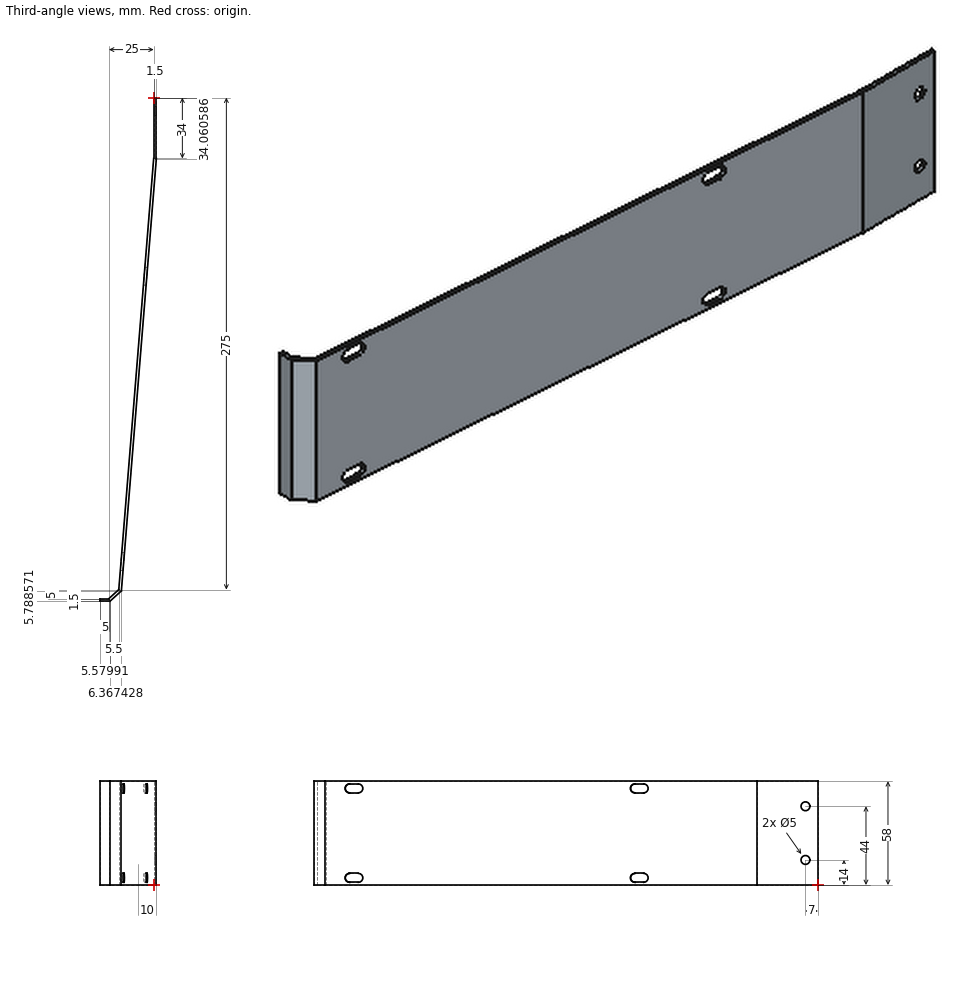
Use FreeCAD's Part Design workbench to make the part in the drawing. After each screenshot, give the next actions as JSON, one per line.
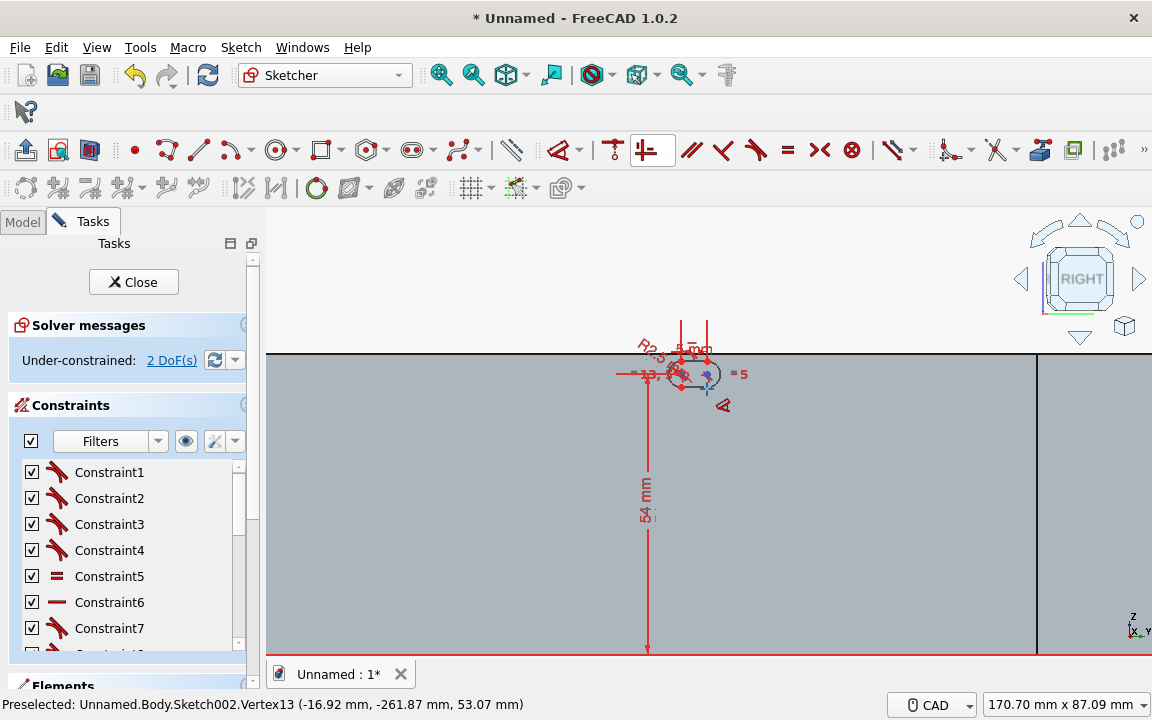
{"action": "left_click", "coordinate": [707, 387]}
{"action": "left_click", "coordinate": [847, 353]}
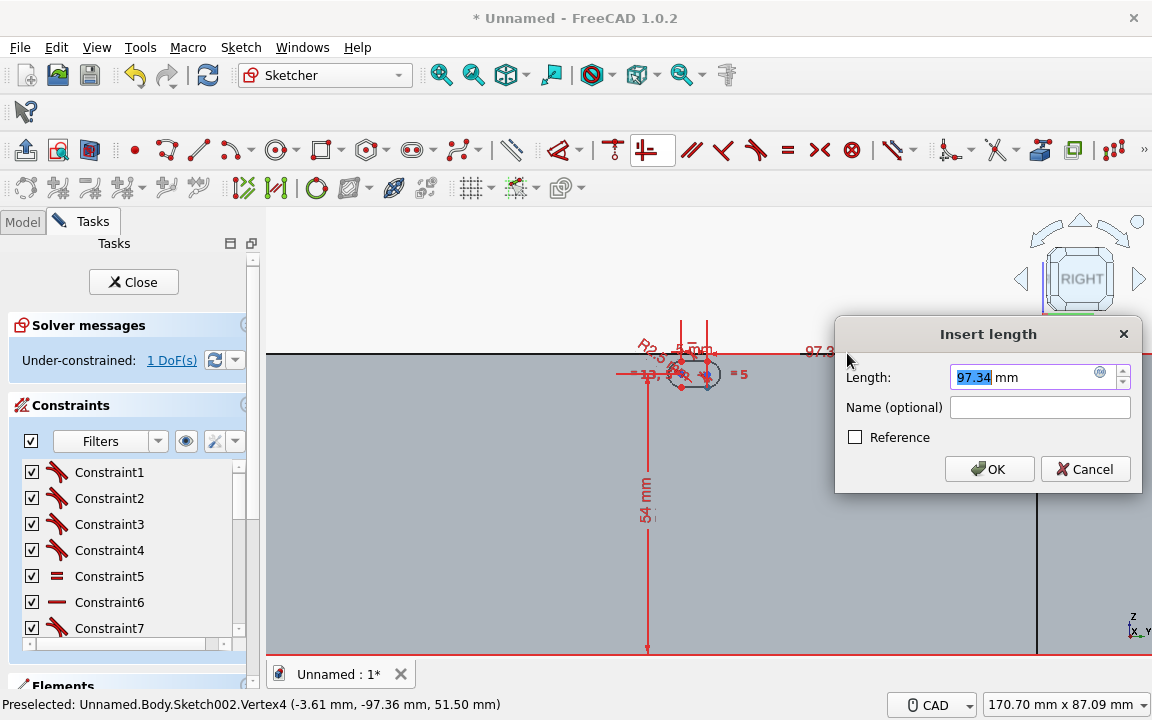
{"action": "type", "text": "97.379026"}
{"action": "key", "text": "Return"}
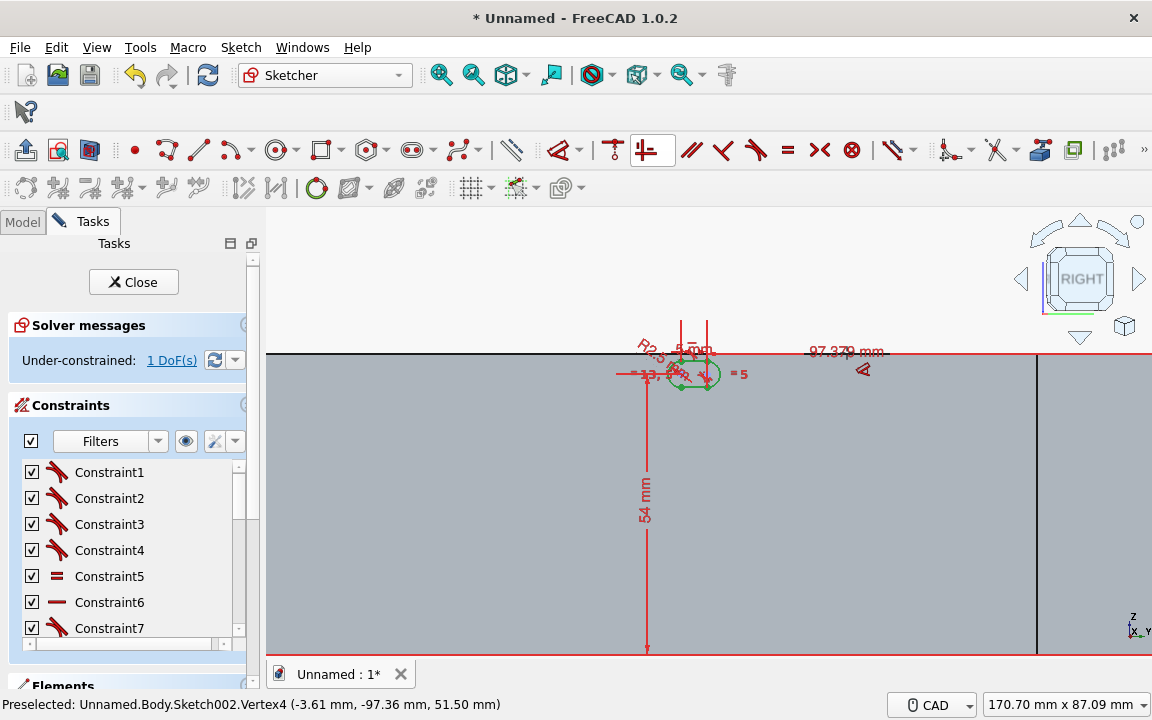
{"action": "scroll", "coordinate": [708, 389], "scroll_direction": "down", "scroll_amount": 5}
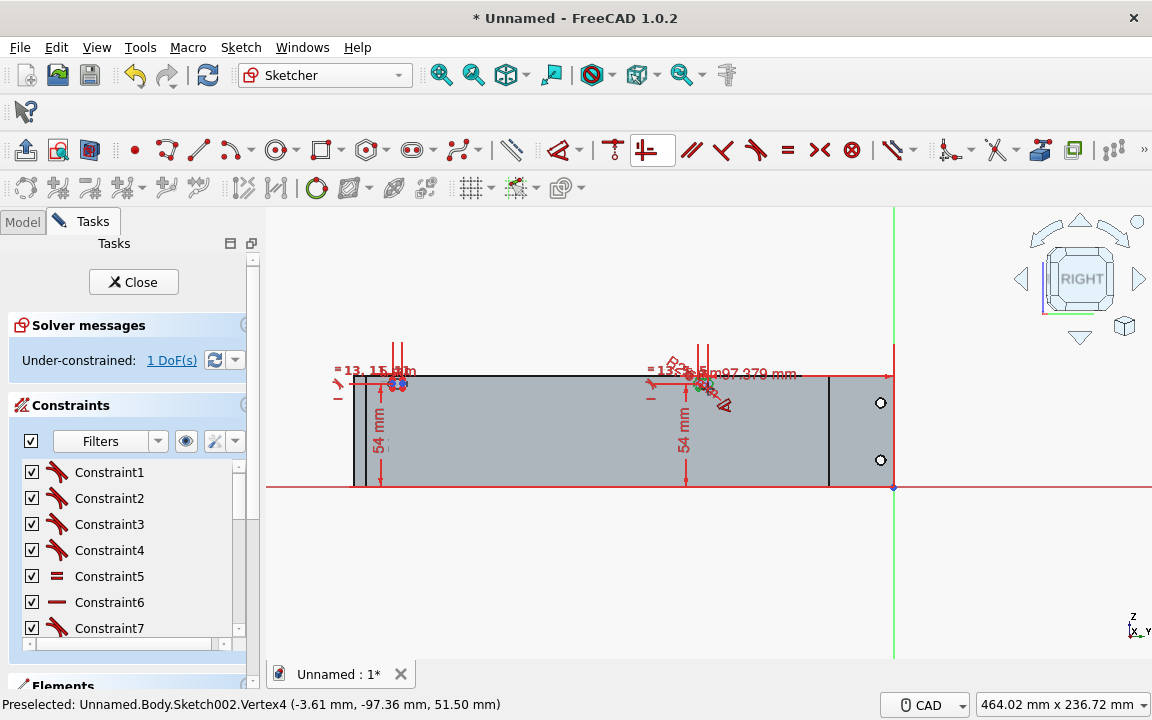
{"action": "scroll", "coordinate": [393, 379], "scroll_direction": "up", "scroll_amount": 5}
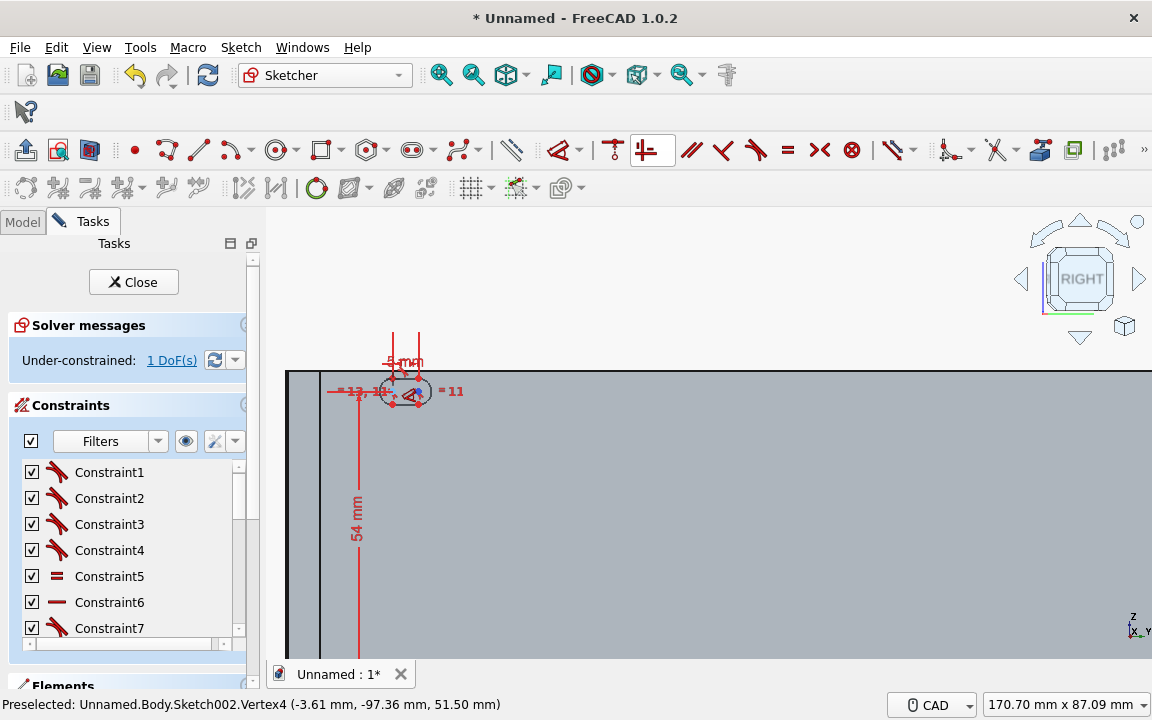
{"action": "left_click", "coordinate": [393, 379]}
{"action": "left_click", "coordinate": [690, 345]}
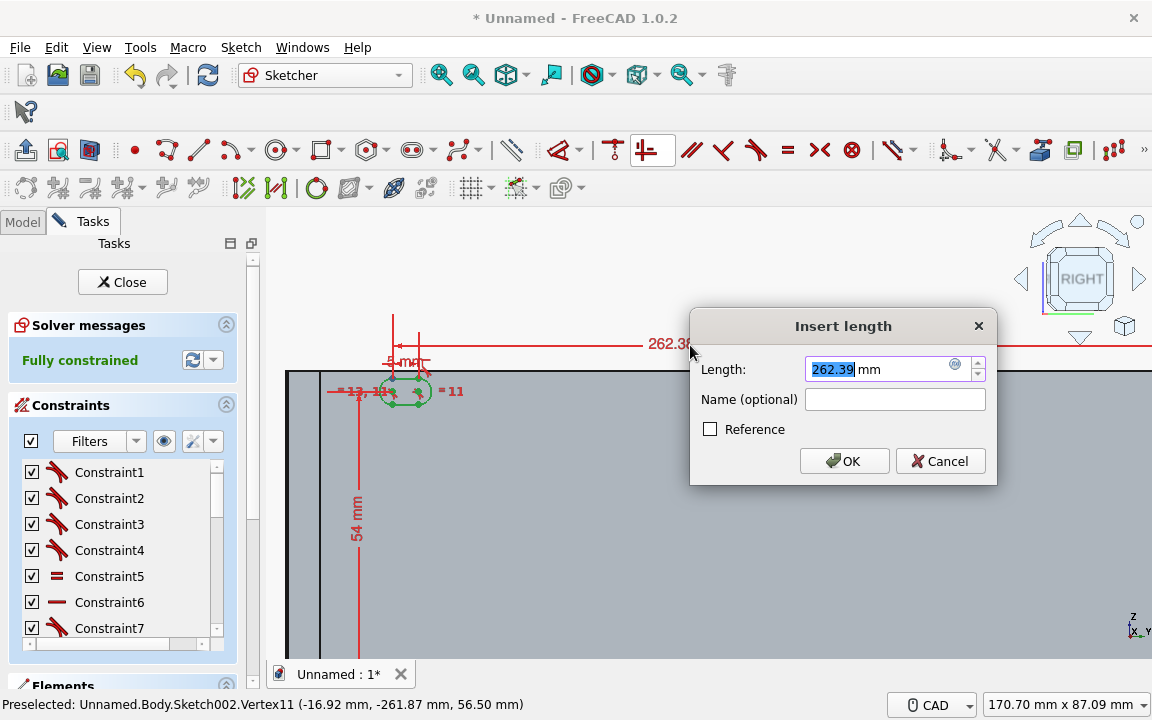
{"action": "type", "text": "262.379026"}
{"action": "key", "text": "Return"}
{"action": "key", "text": "Escape"}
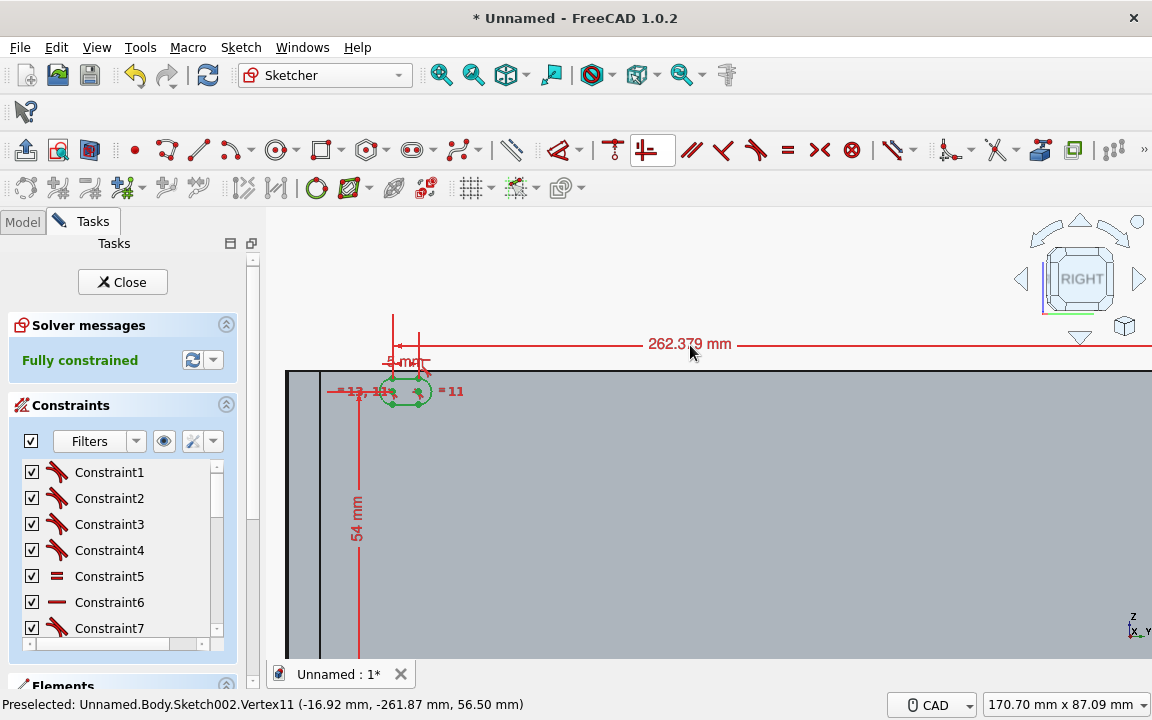
{"action": "left_click", "coordinate": [123, 282]}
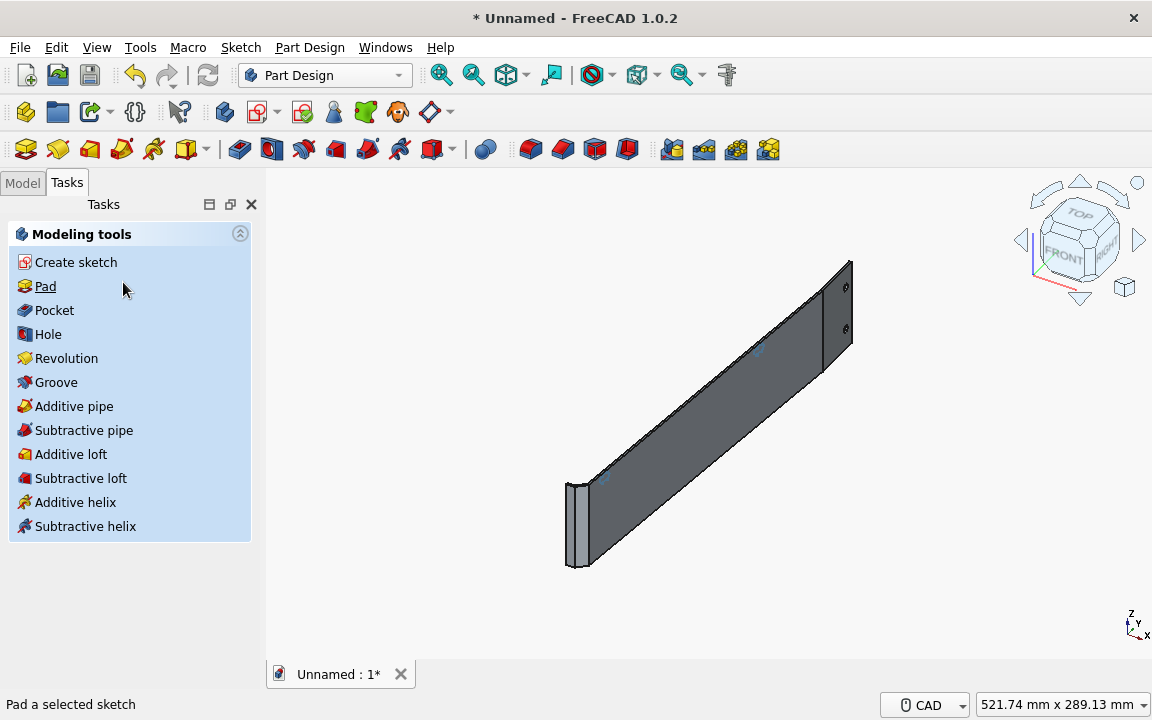
{"action": "left_click", "coordinate": [240, 150]}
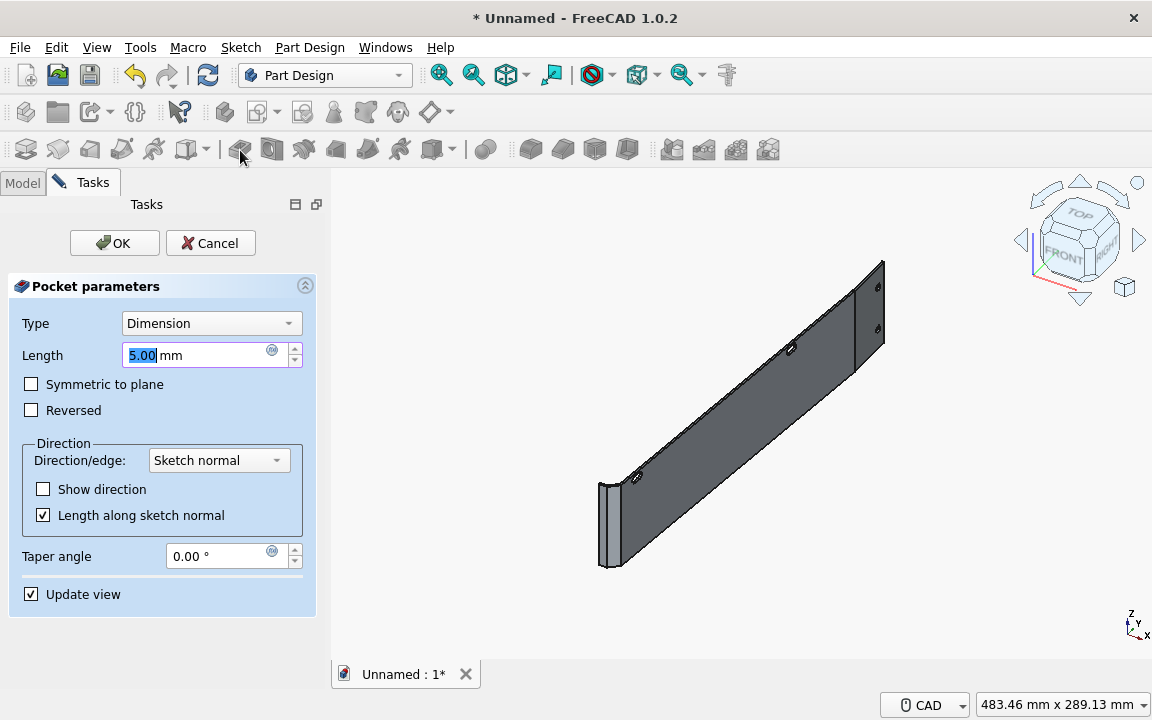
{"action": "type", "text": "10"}
{"action": "key", "text": "Tab"}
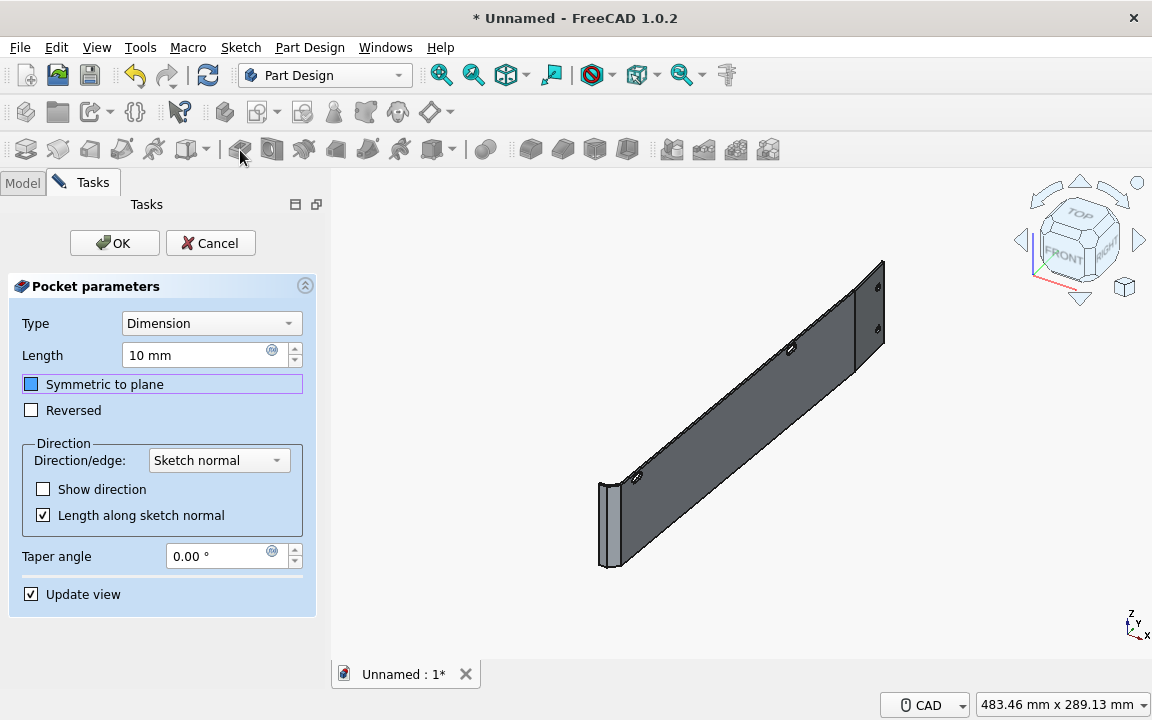
{"action": "left_click", "coordinate": [115, 243]}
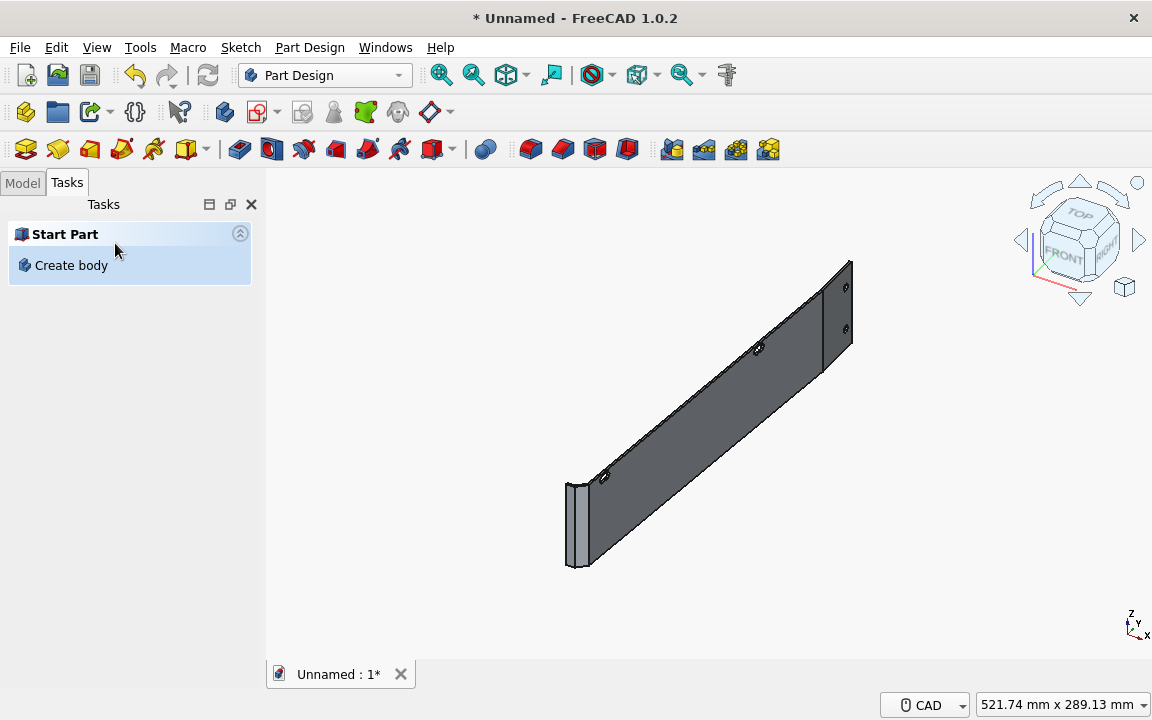
{"action": "left_click", "coordinate": [23, 182]}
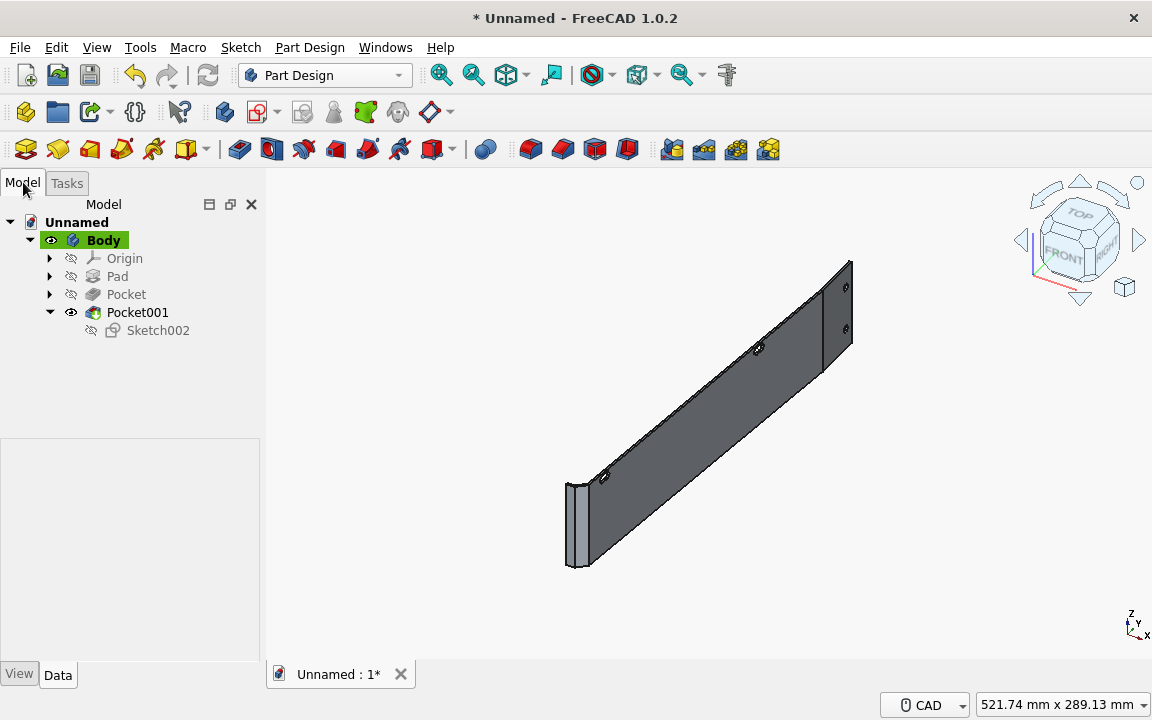
{"action": "left_click", "coordinate": [50, 258]}